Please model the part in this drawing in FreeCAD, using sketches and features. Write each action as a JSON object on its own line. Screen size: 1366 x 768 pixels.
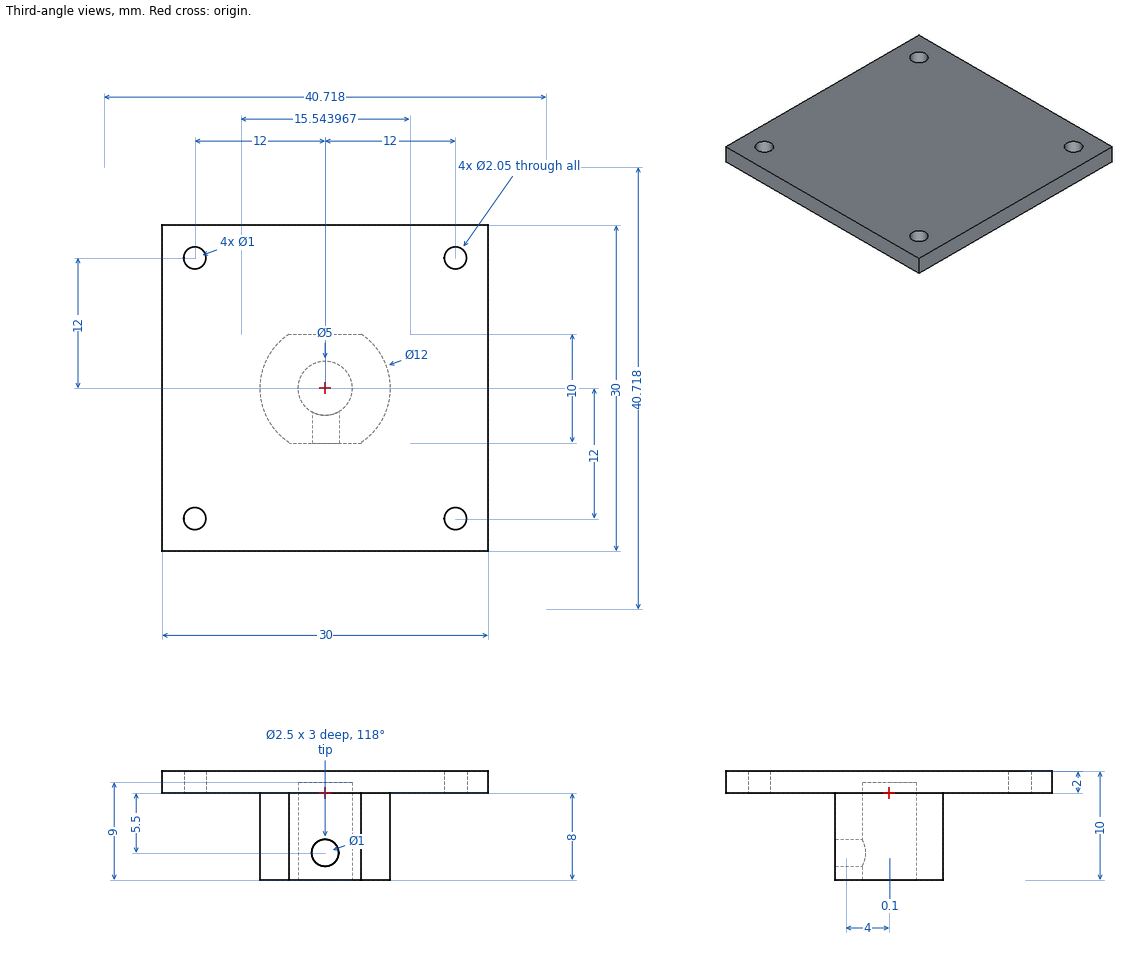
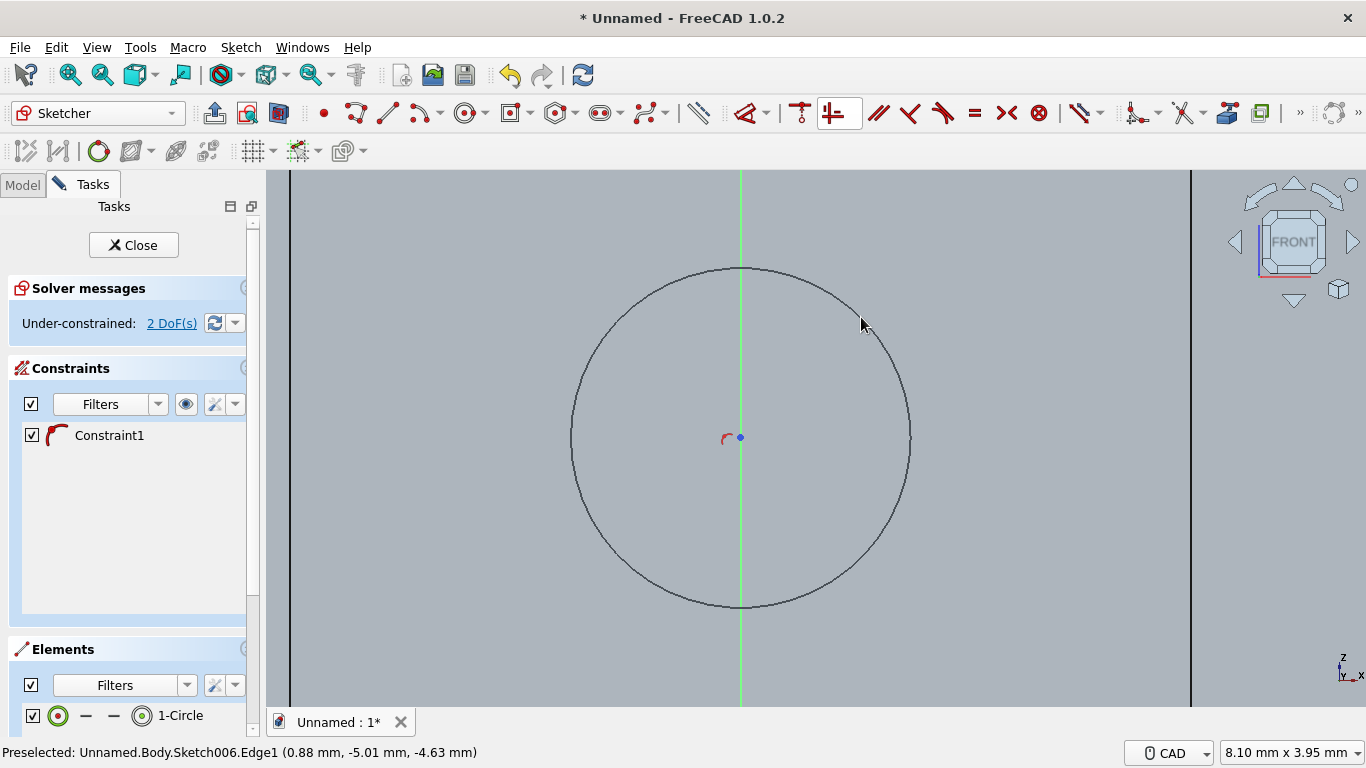
{"action": "left_click", "coordinate": [746, 114]}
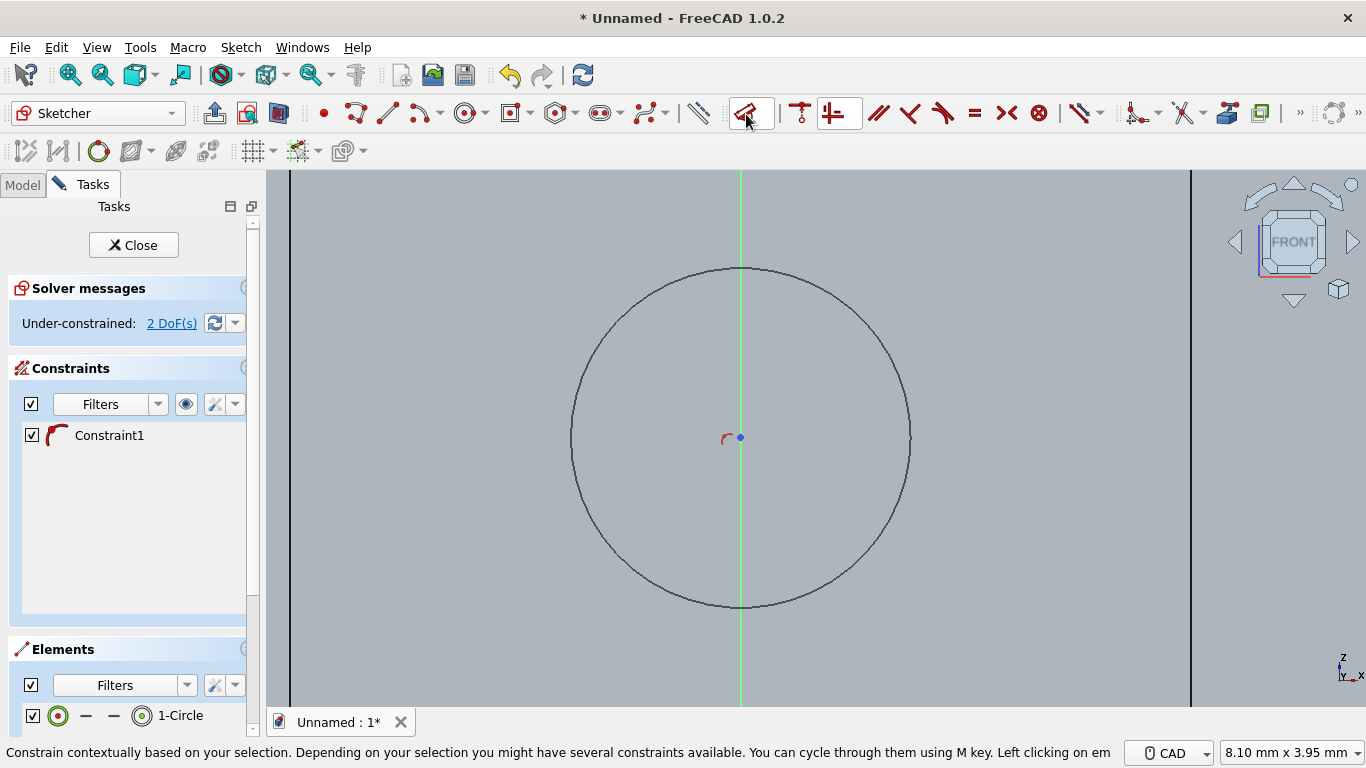
{"action": "left_click", "coordinate": [861, 318]}
{"action": "left_click", "coordinate": [884, 295]}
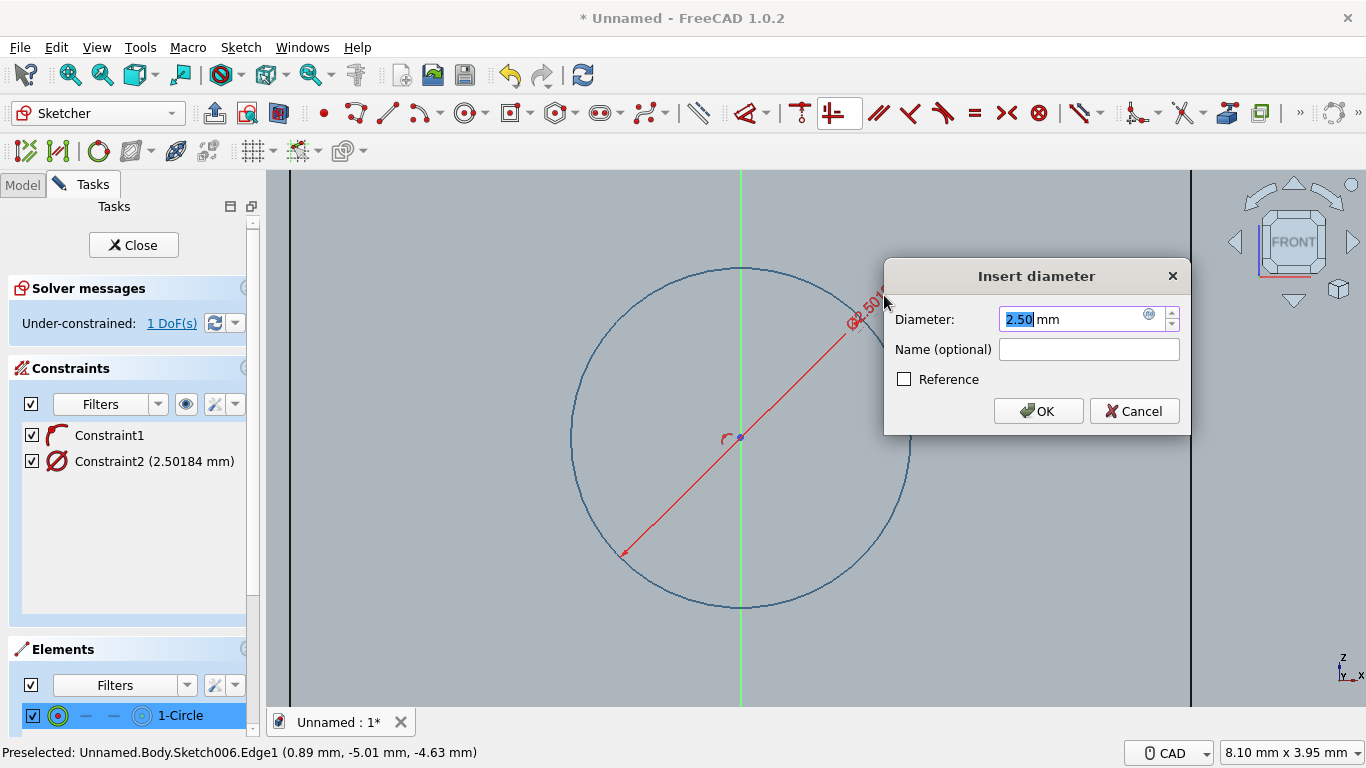
{"action": "type", "text": "2.5"}
{"action": "key", "text": "Return"}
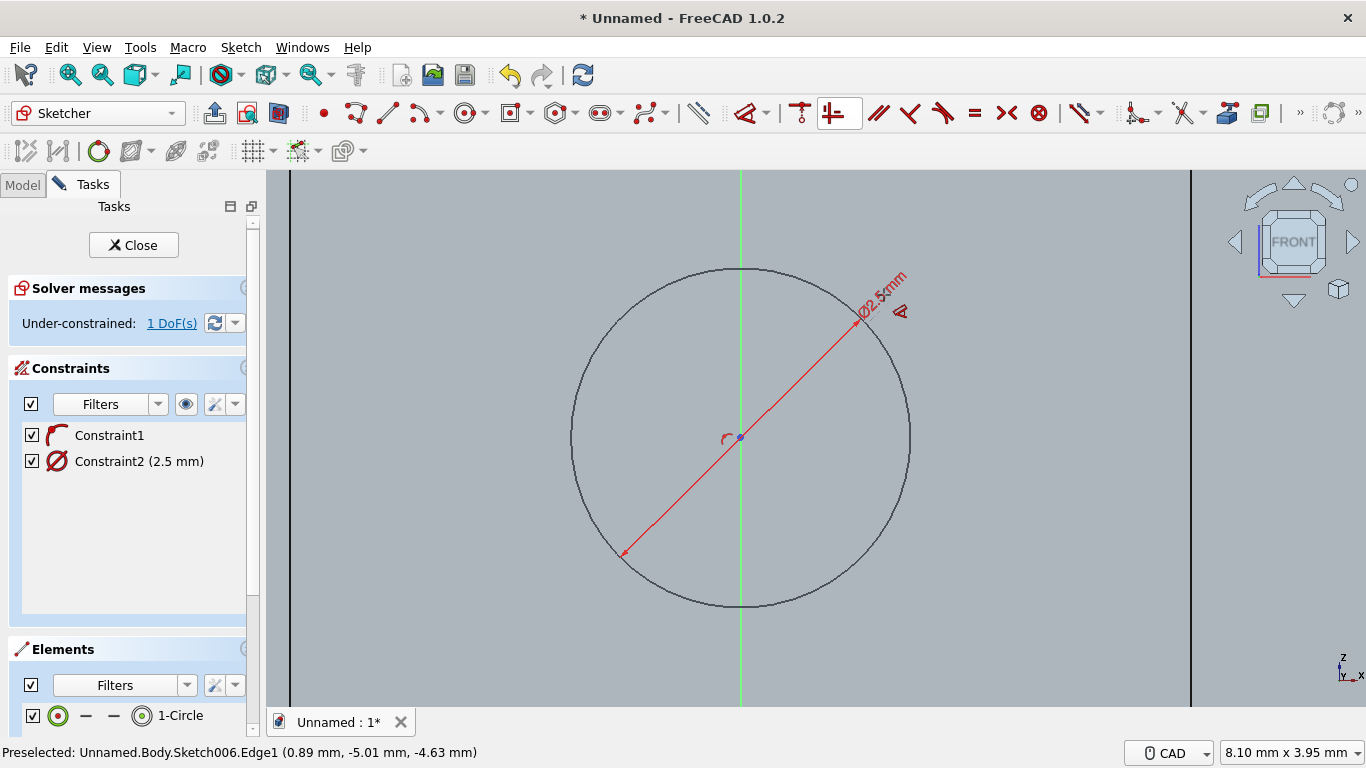
{"action": "left_click", "coordinate": [741, 438]}
{"action": "left_click", "coordinate": [775, 318]}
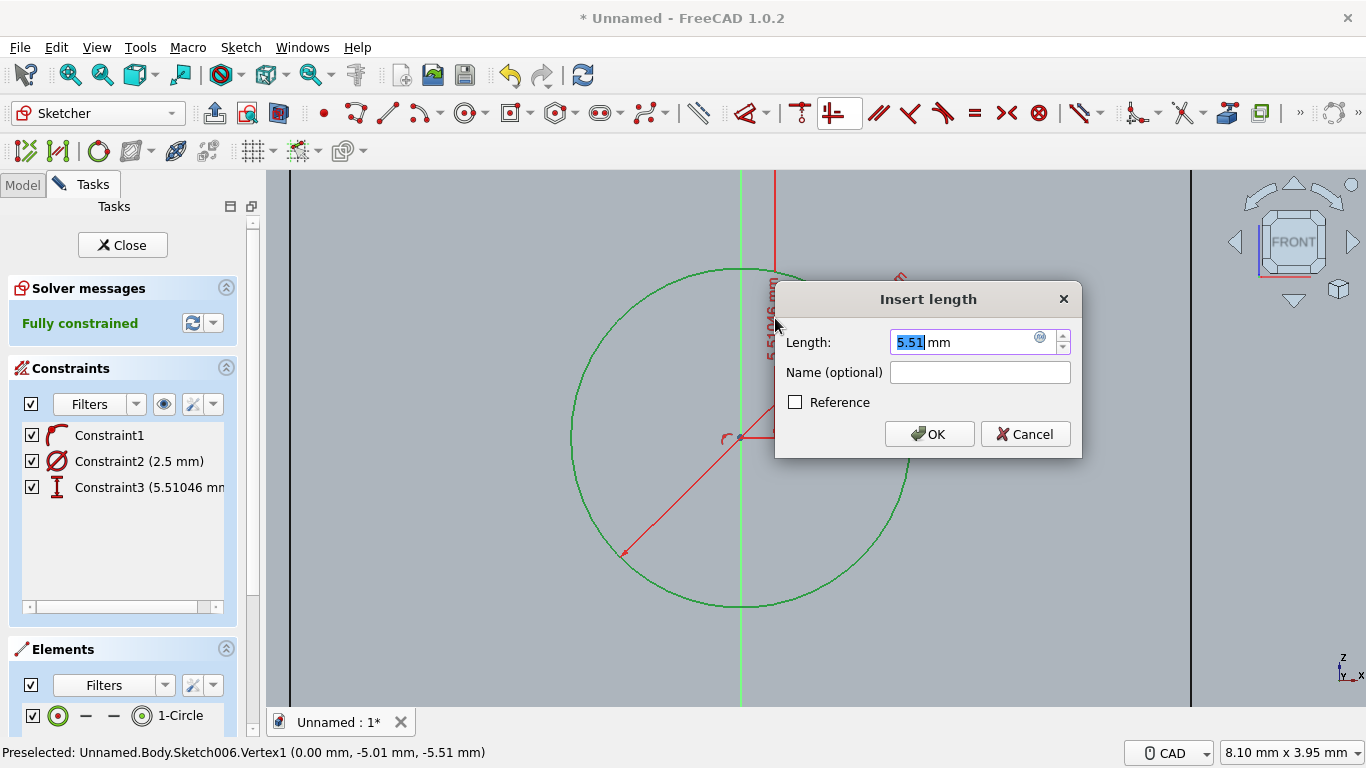
{"action": "type", "text": "5.5"}
{"action": "key", "text": "Return"}
{"action": "key", "text": "Escape"}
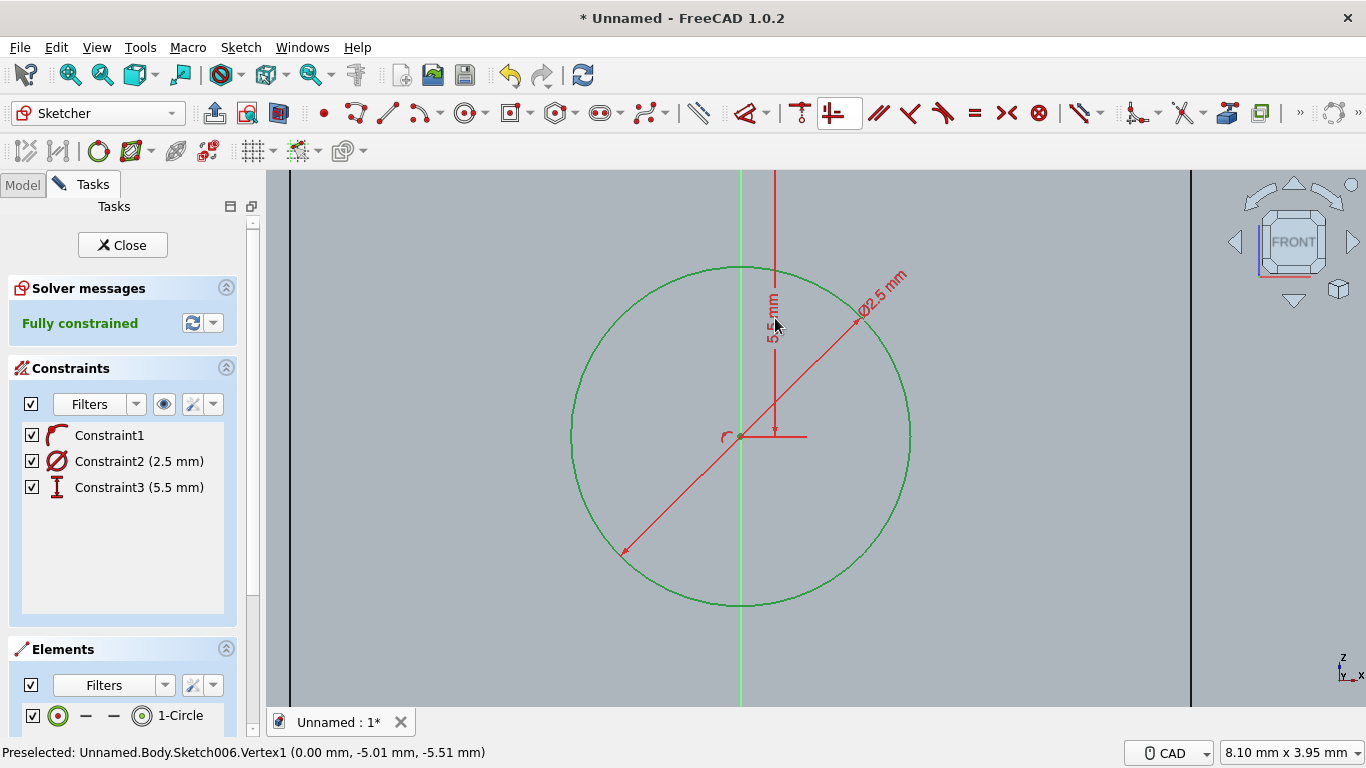
{"action": "left_click", "coordinate": [123, 245]}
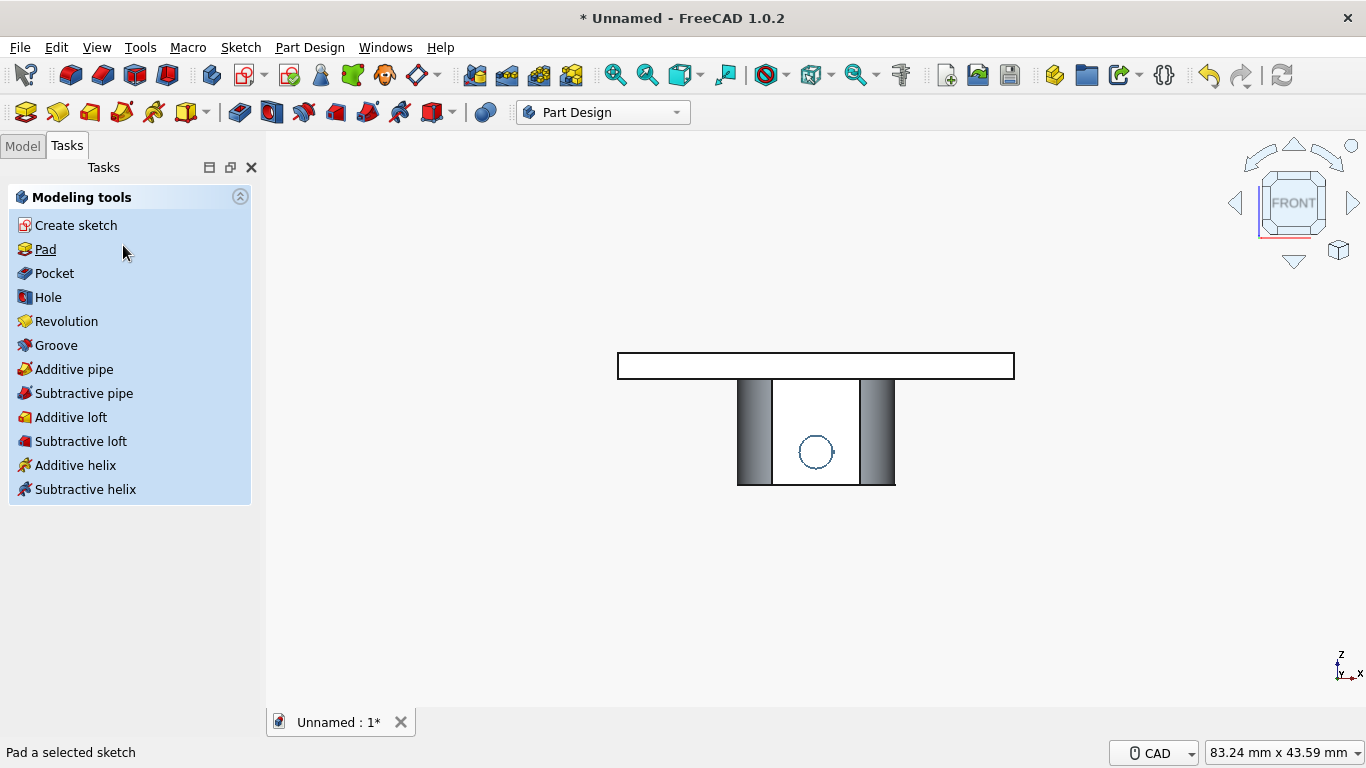
{"action": "left_click", "coordinate": [272, 112]}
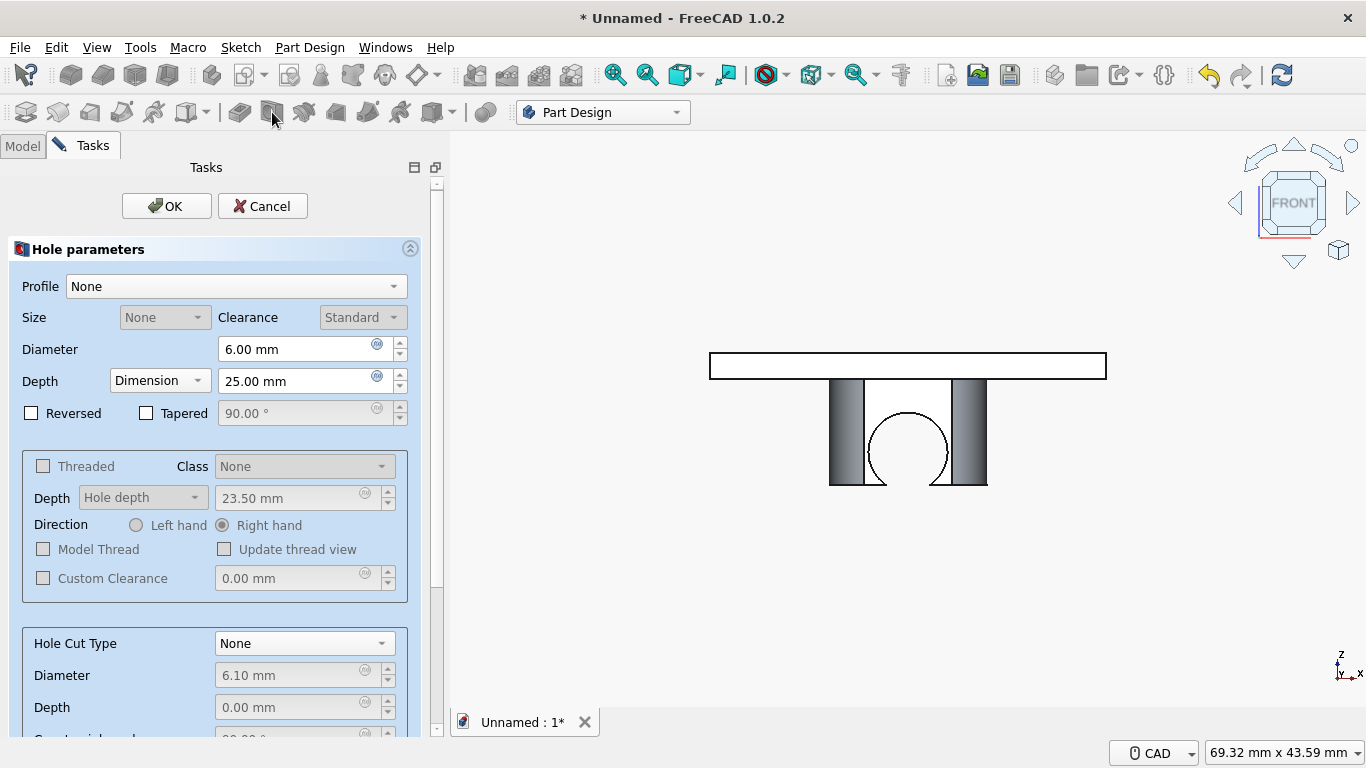
{"action": "triple_click", "coordinate": [305, 349]}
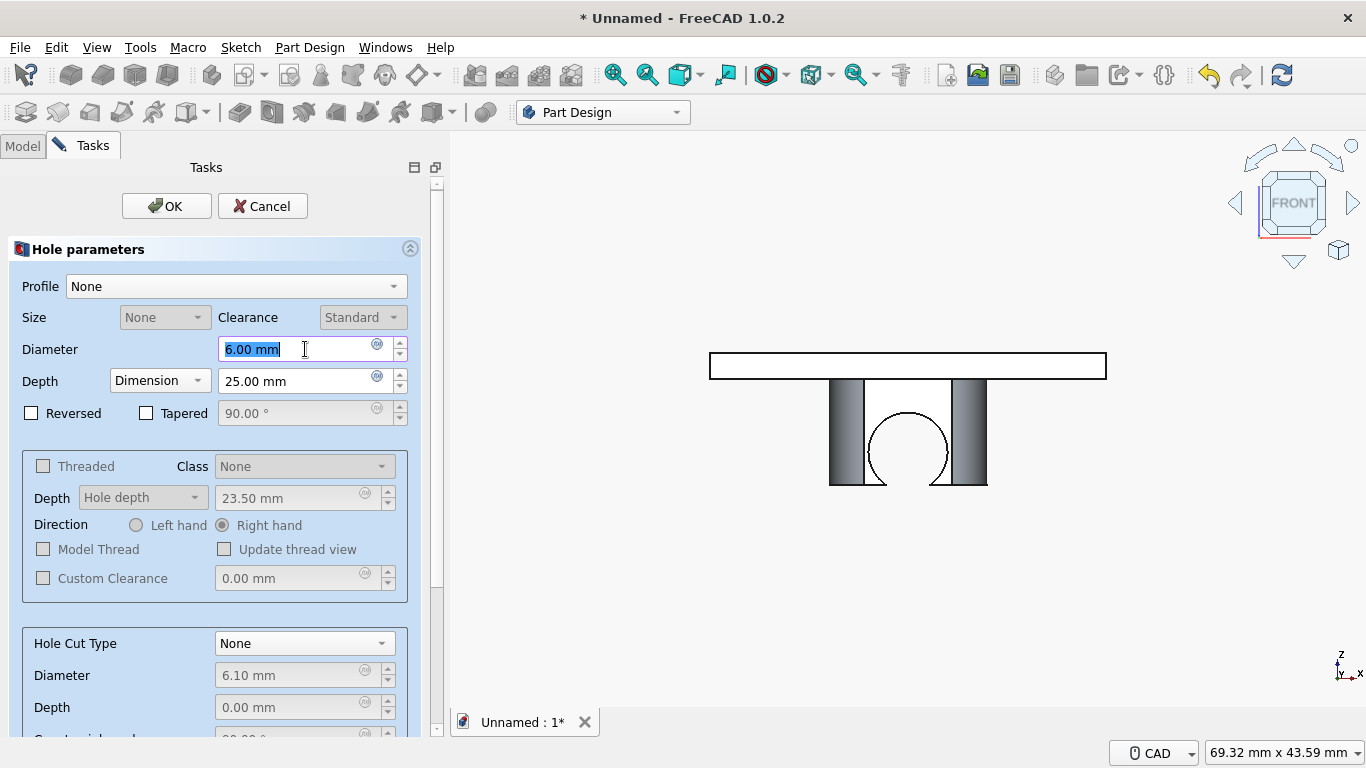
{"action": "type", "text": "2.5"}
{"action": "key", "text": "Tab"}